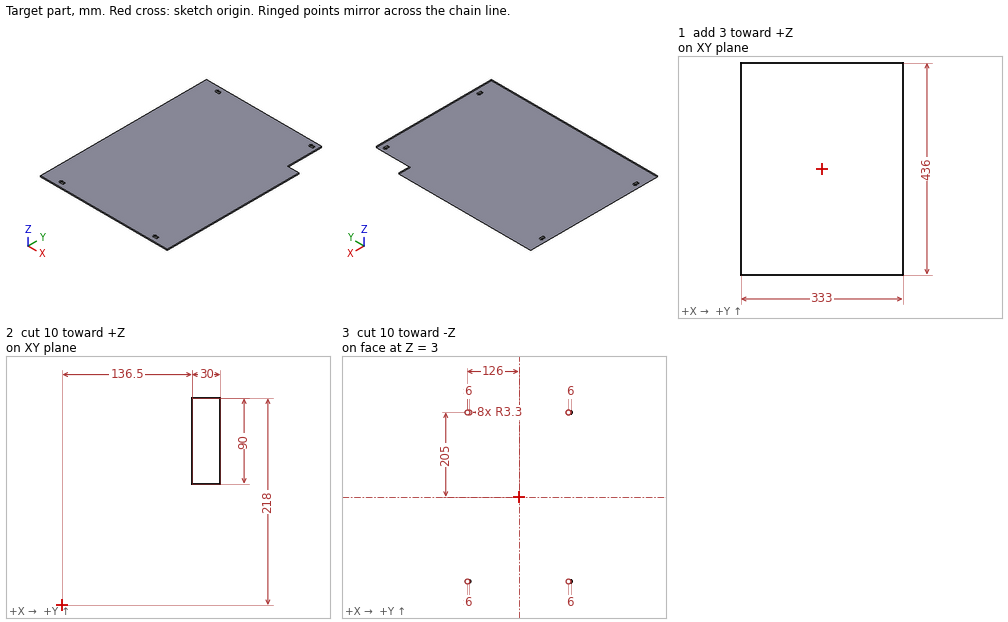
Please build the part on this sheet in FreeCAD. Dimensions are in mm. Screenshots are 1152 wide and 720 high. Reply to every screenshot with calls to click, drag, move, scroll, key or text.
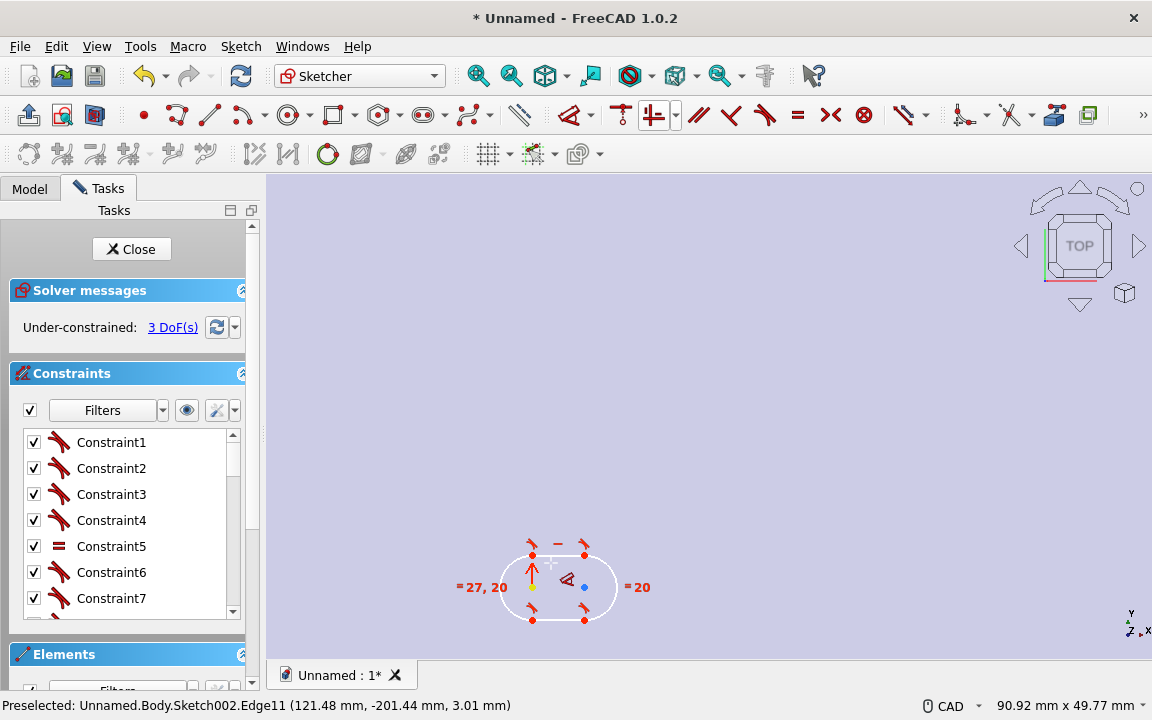
click(548, 556)
click(559, 590)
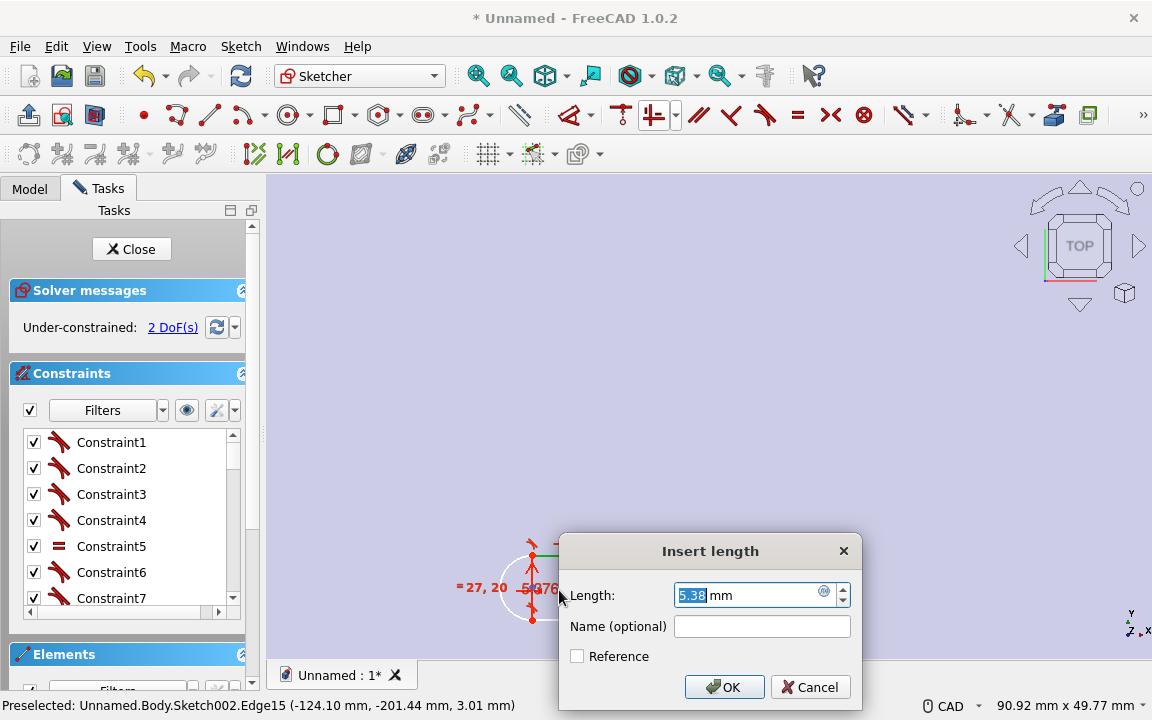
text(6)
key(Return)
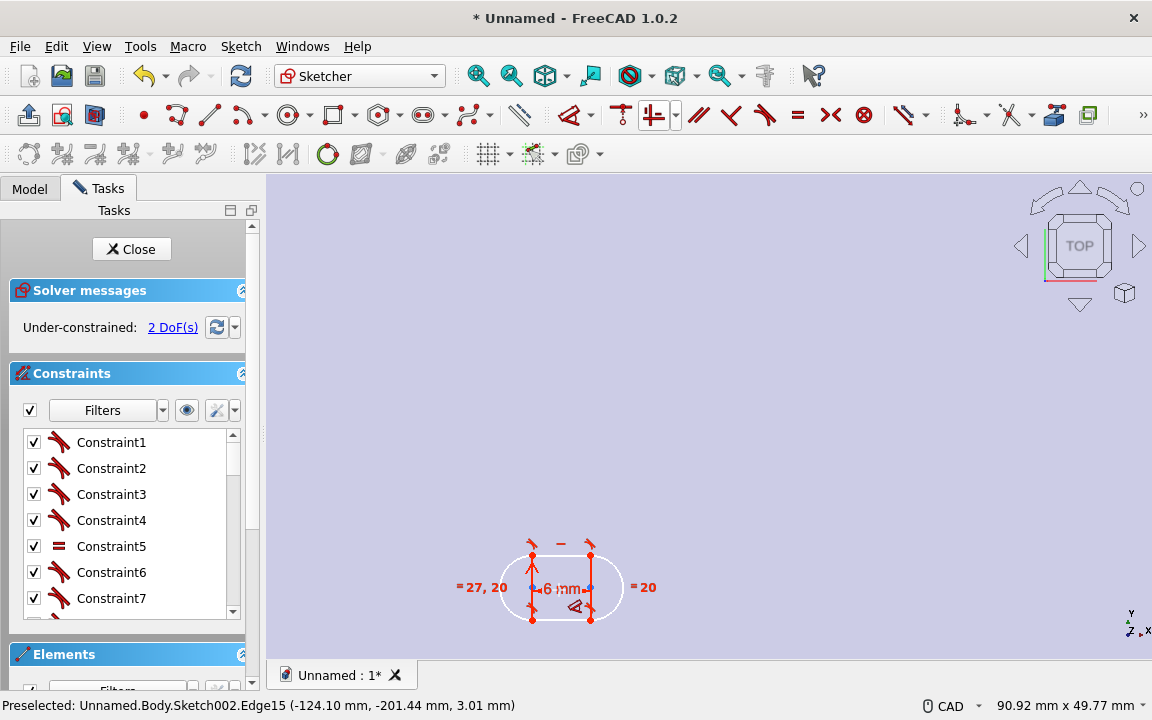
scroll(551, 563, down, 13)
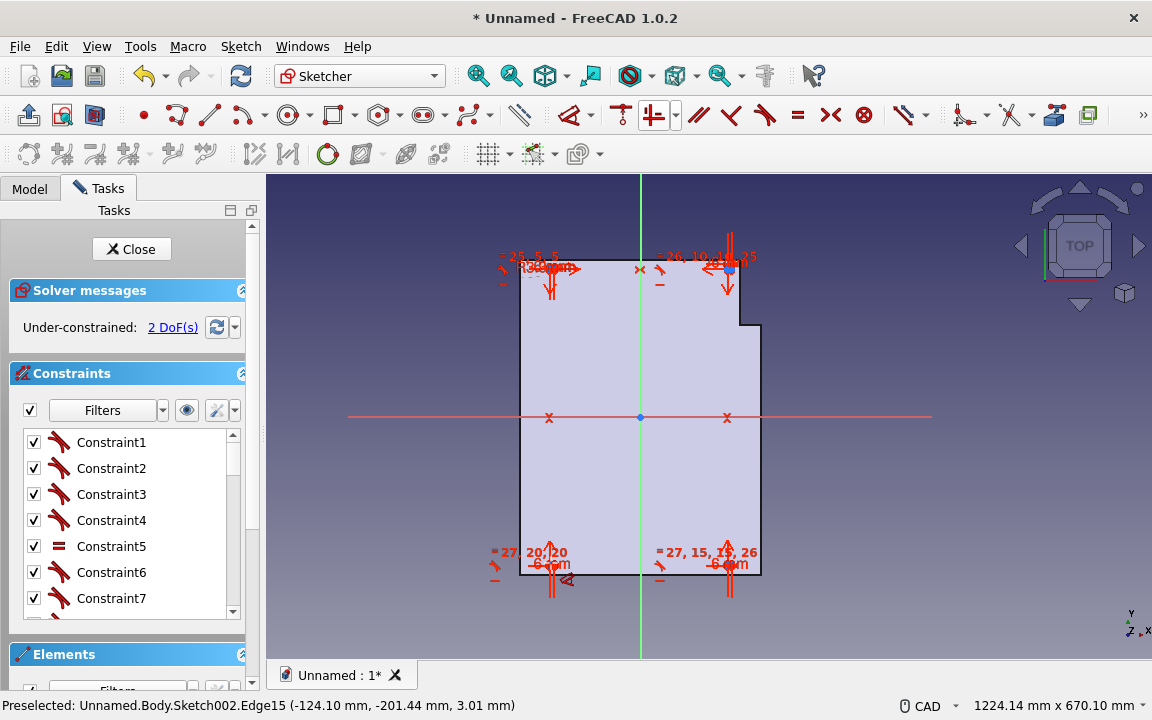
scroll(550, 267, up, 9)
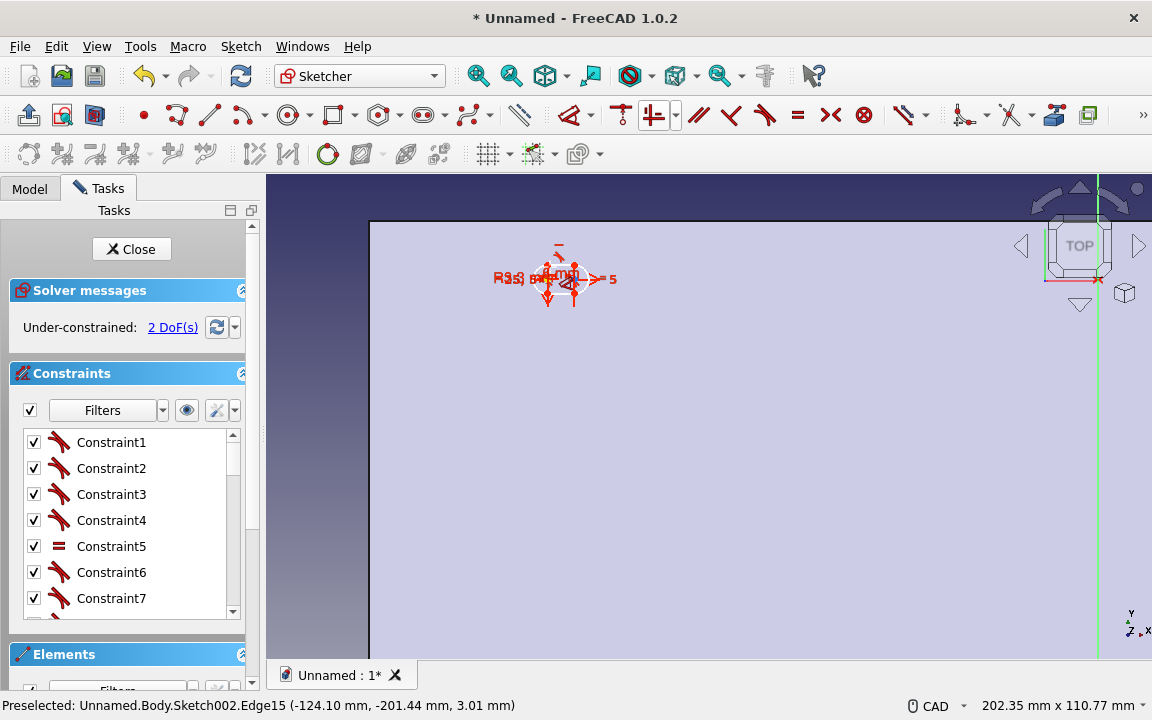
click(548, 265)
click(767, 231)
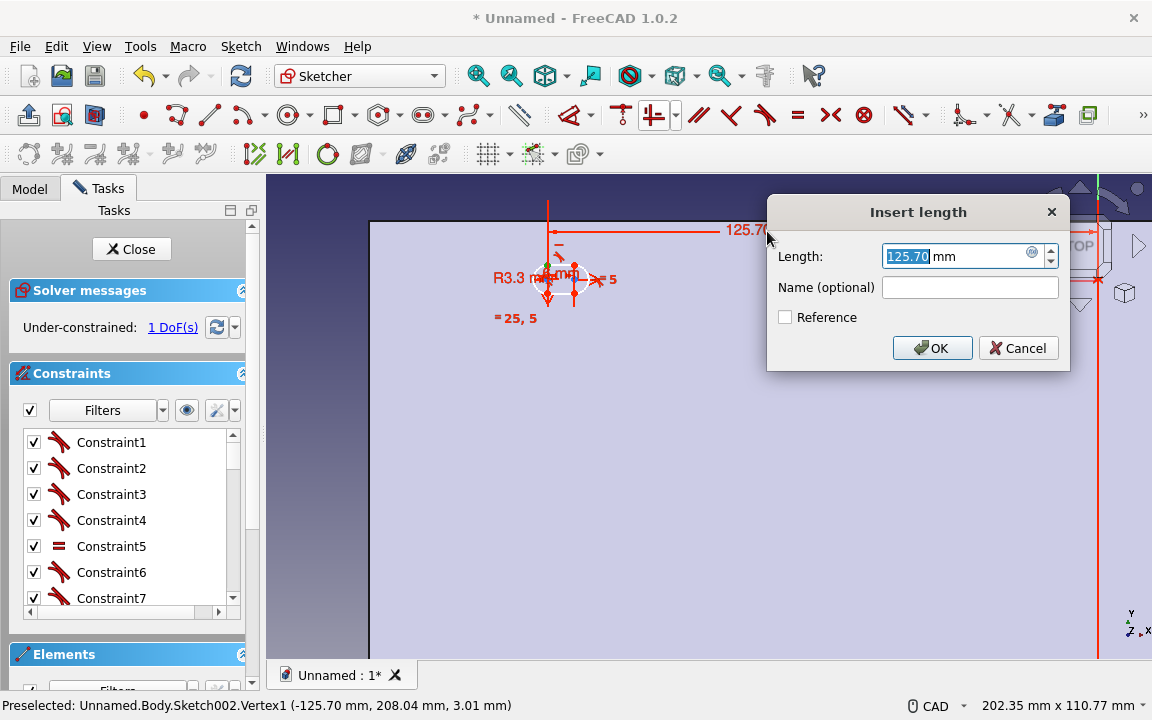
text(126)
key(Return)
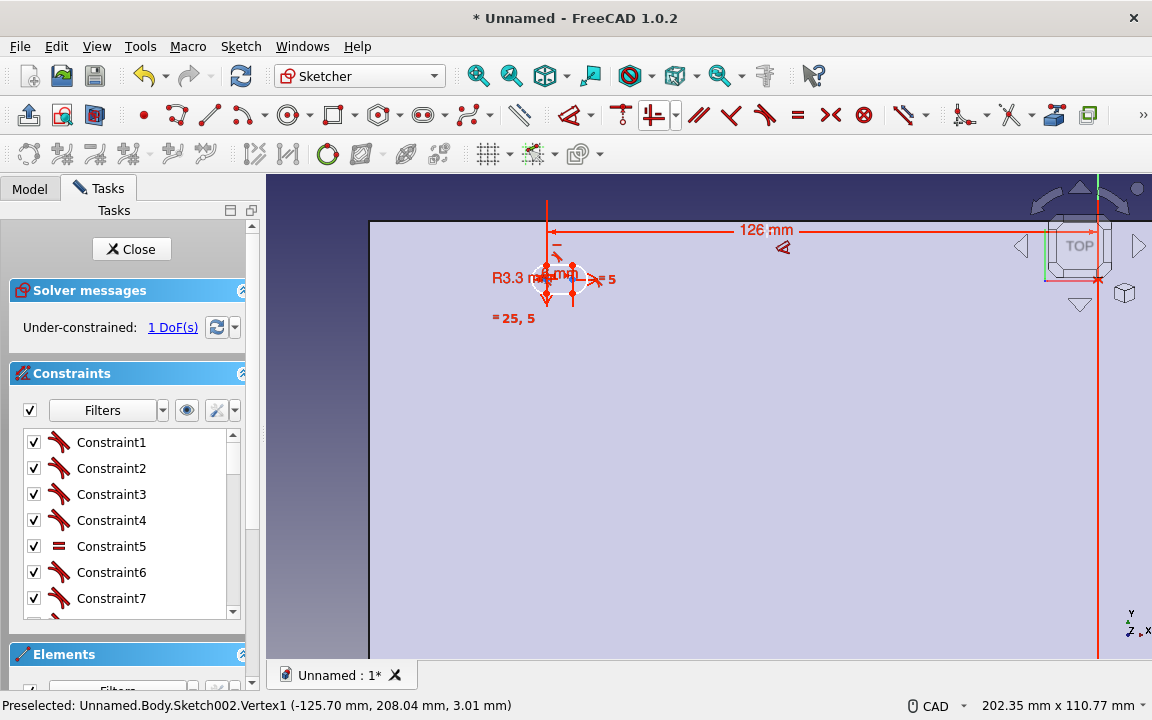
click(547, 280)
click(513, 455)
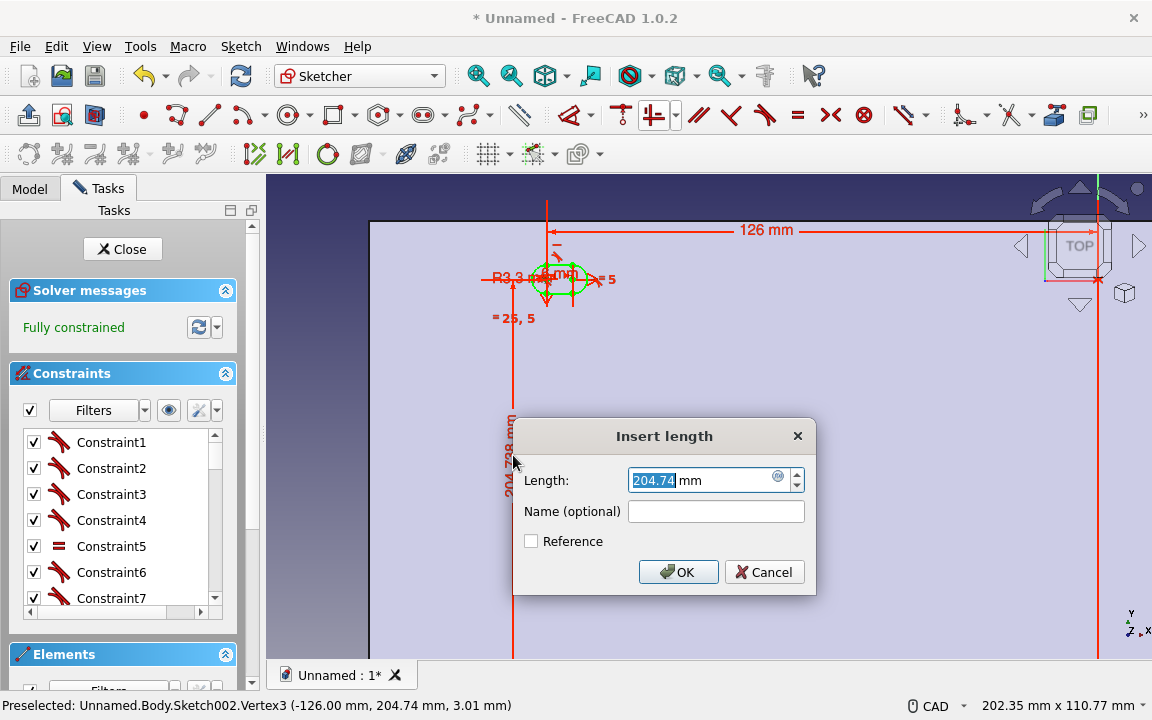
text(205)
key(Return)
key(Escape)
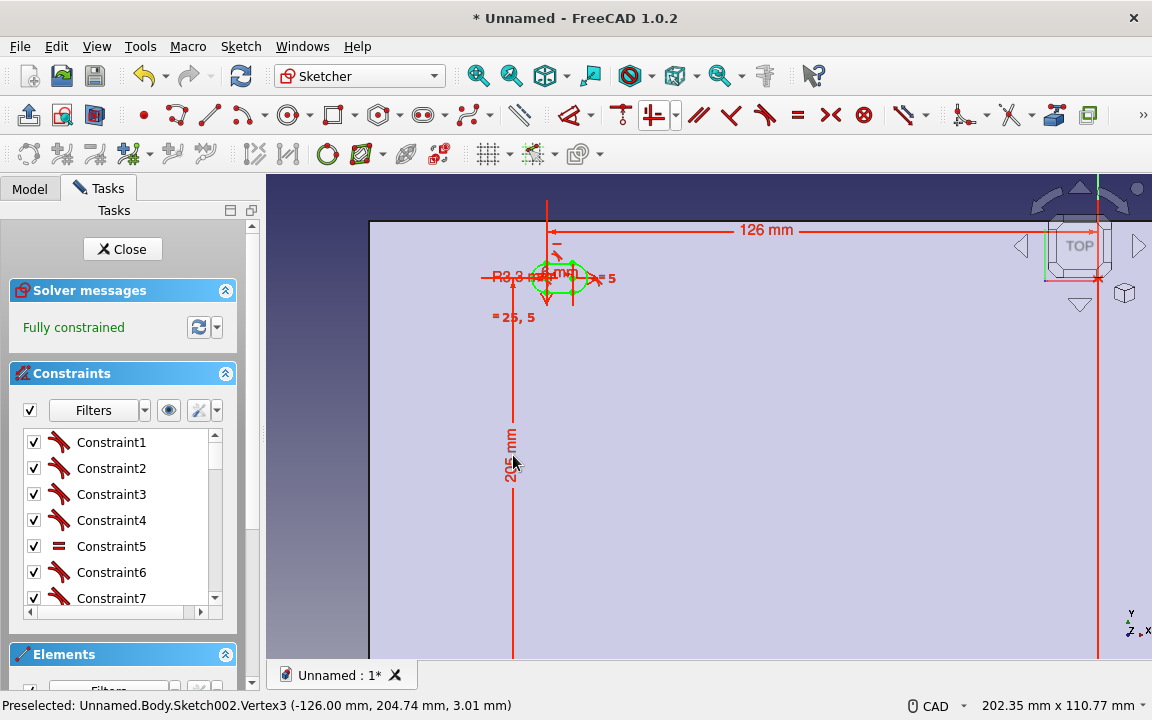
click(123, 249)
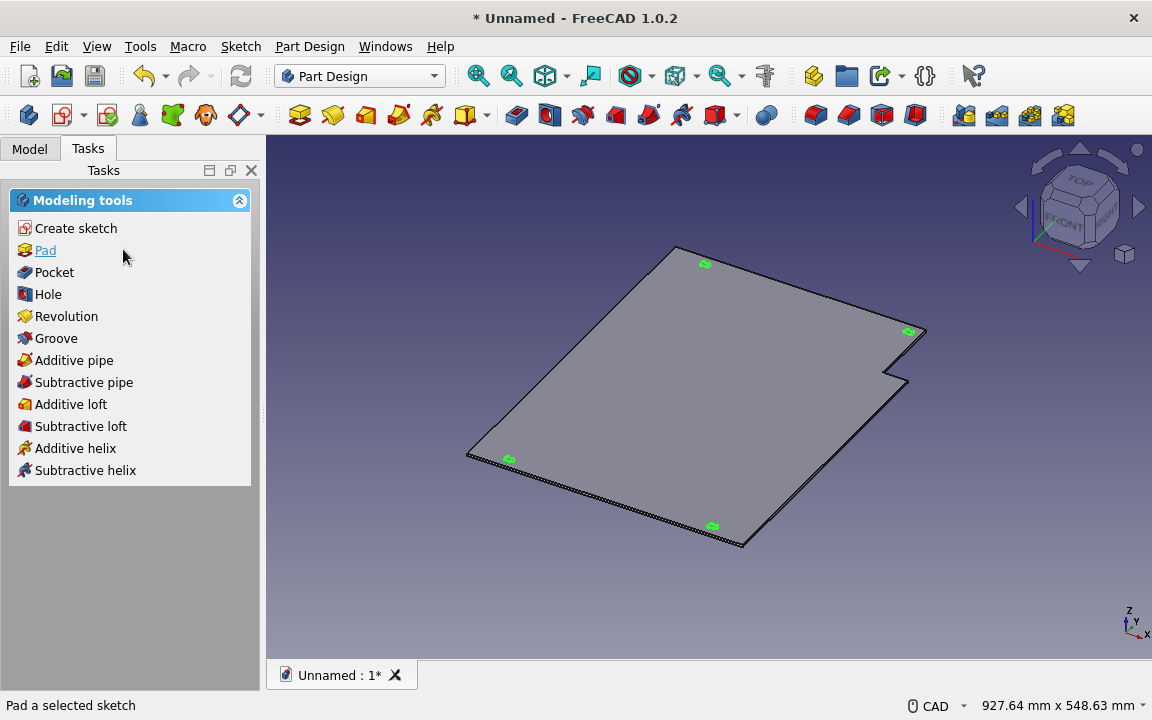
click(517, 116)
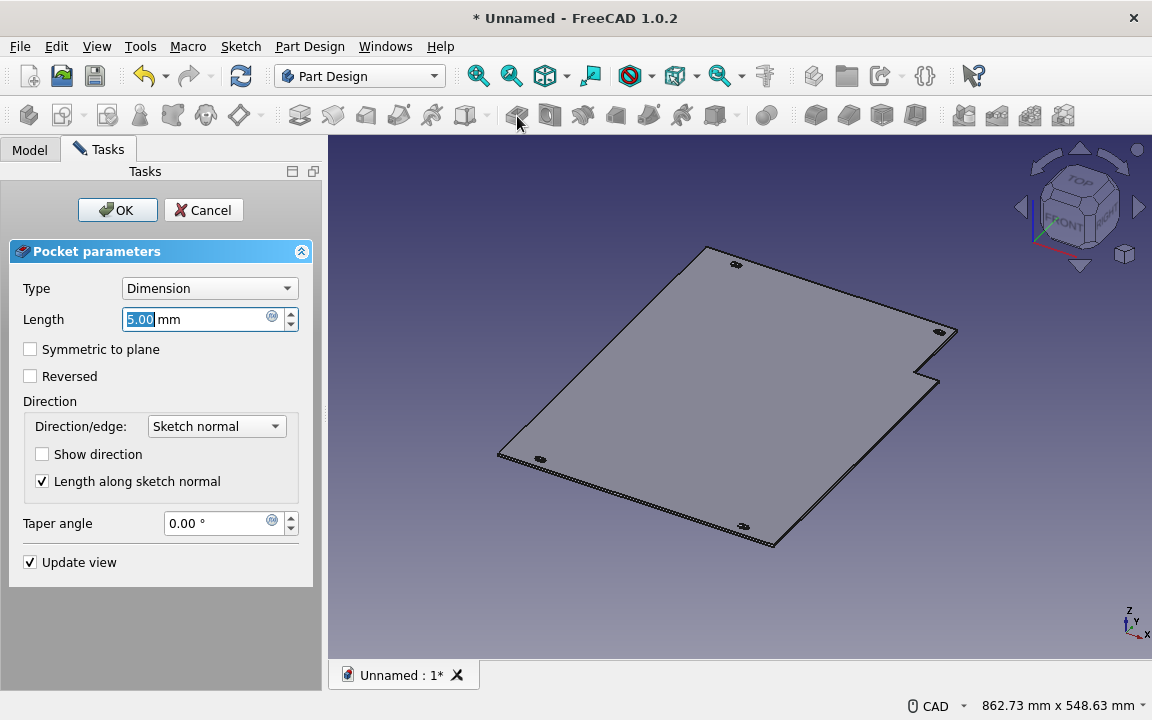
text(10)
key(Tab)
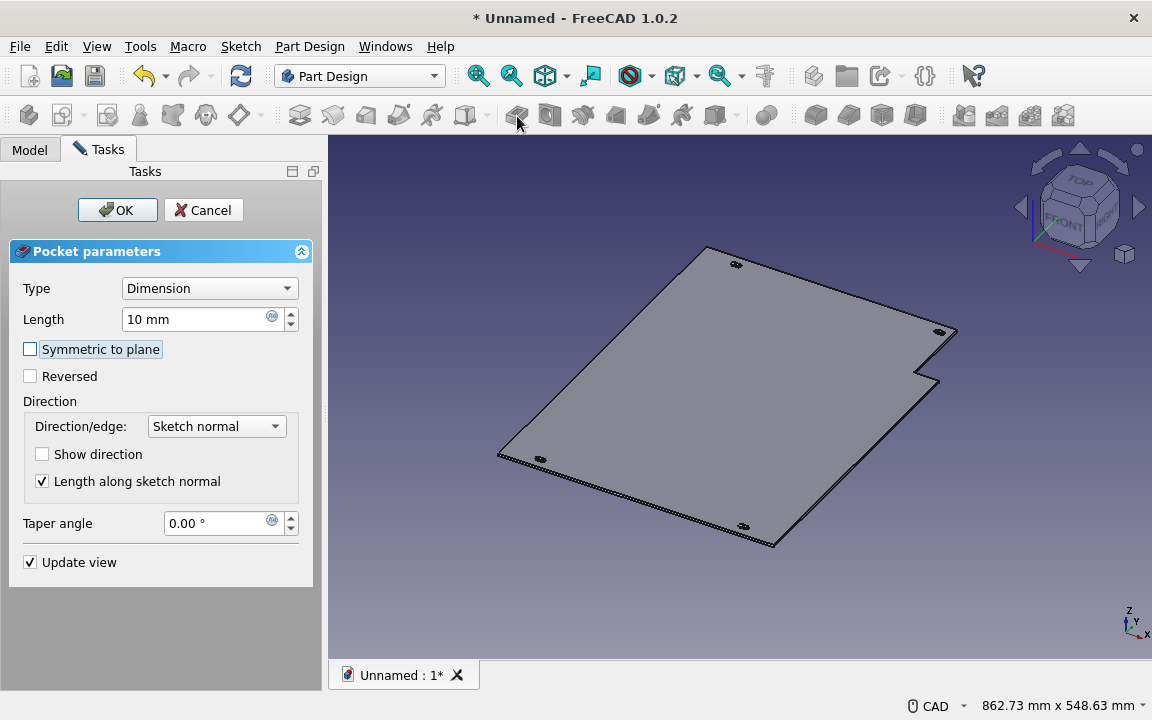
click(118, 210)